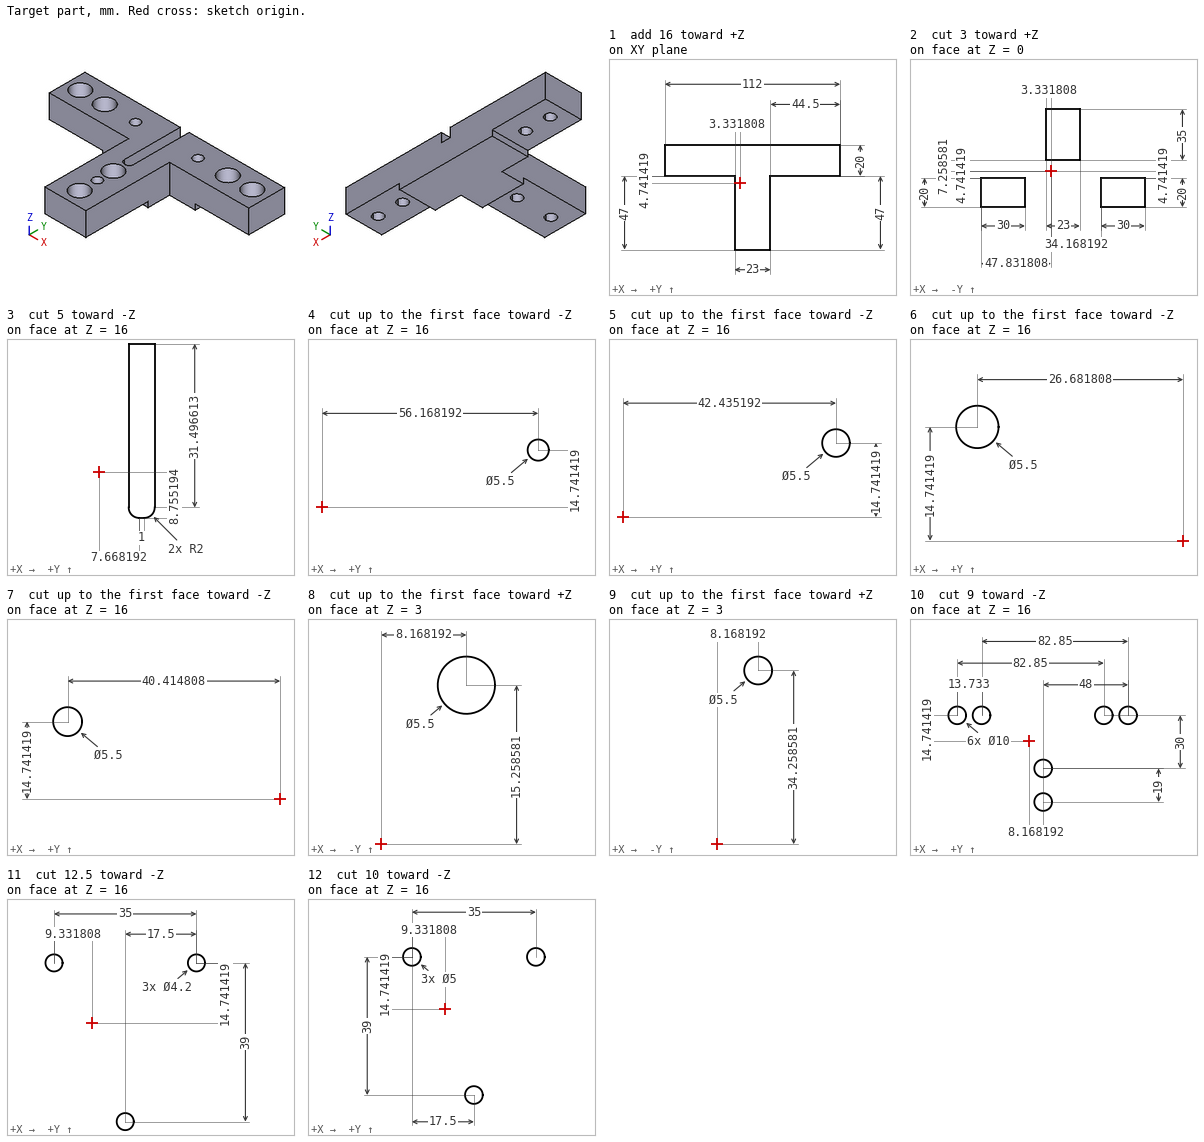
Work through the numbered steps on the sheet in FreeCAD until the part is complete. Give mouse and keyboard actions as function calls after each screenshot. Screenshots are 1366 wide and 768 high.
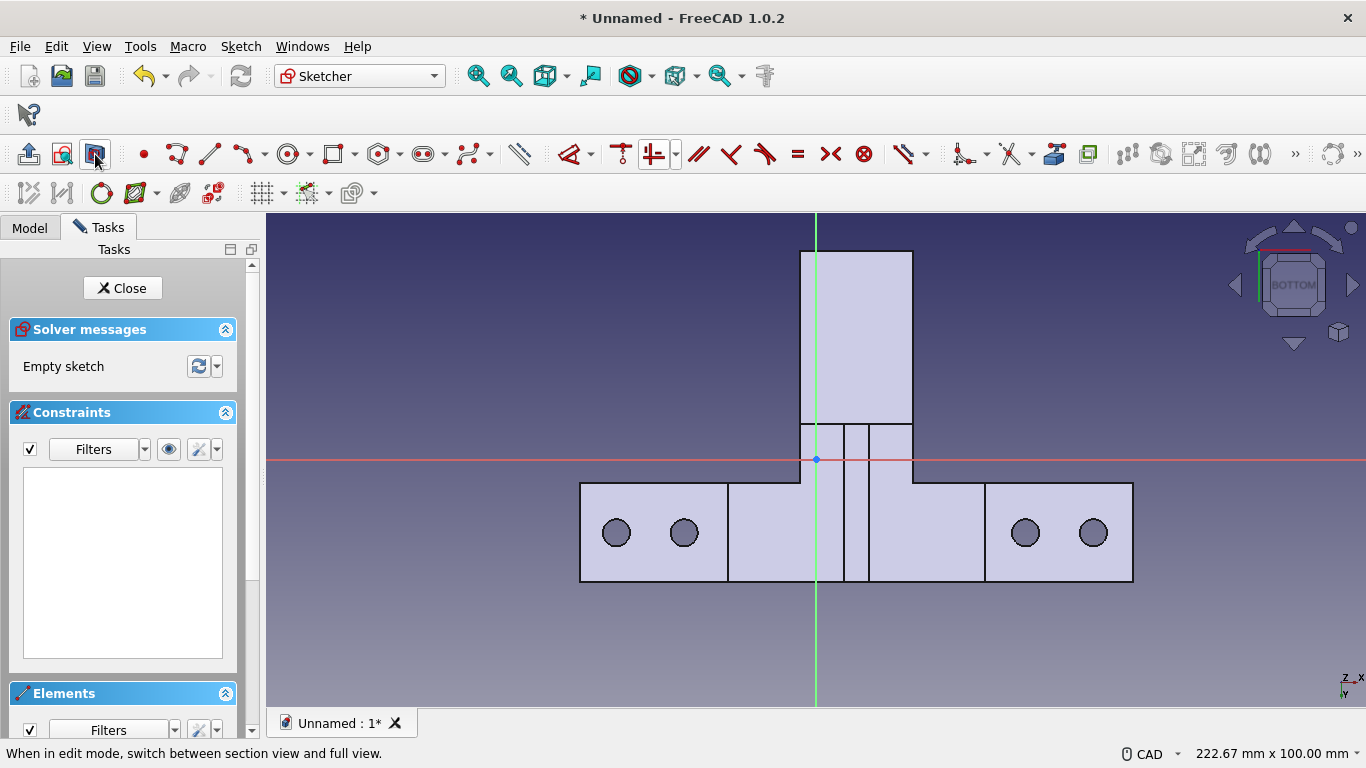
scroll(867, 377, up, 12)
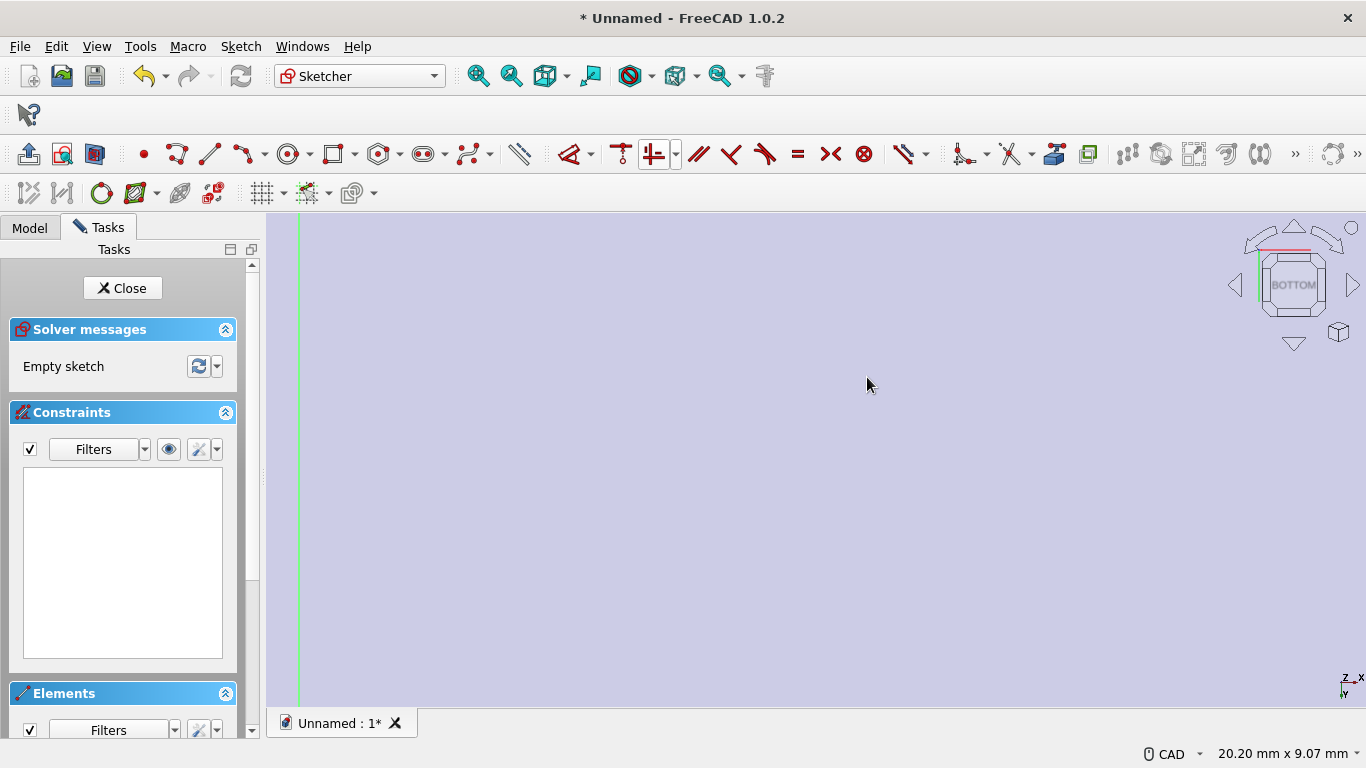
click(288, 154)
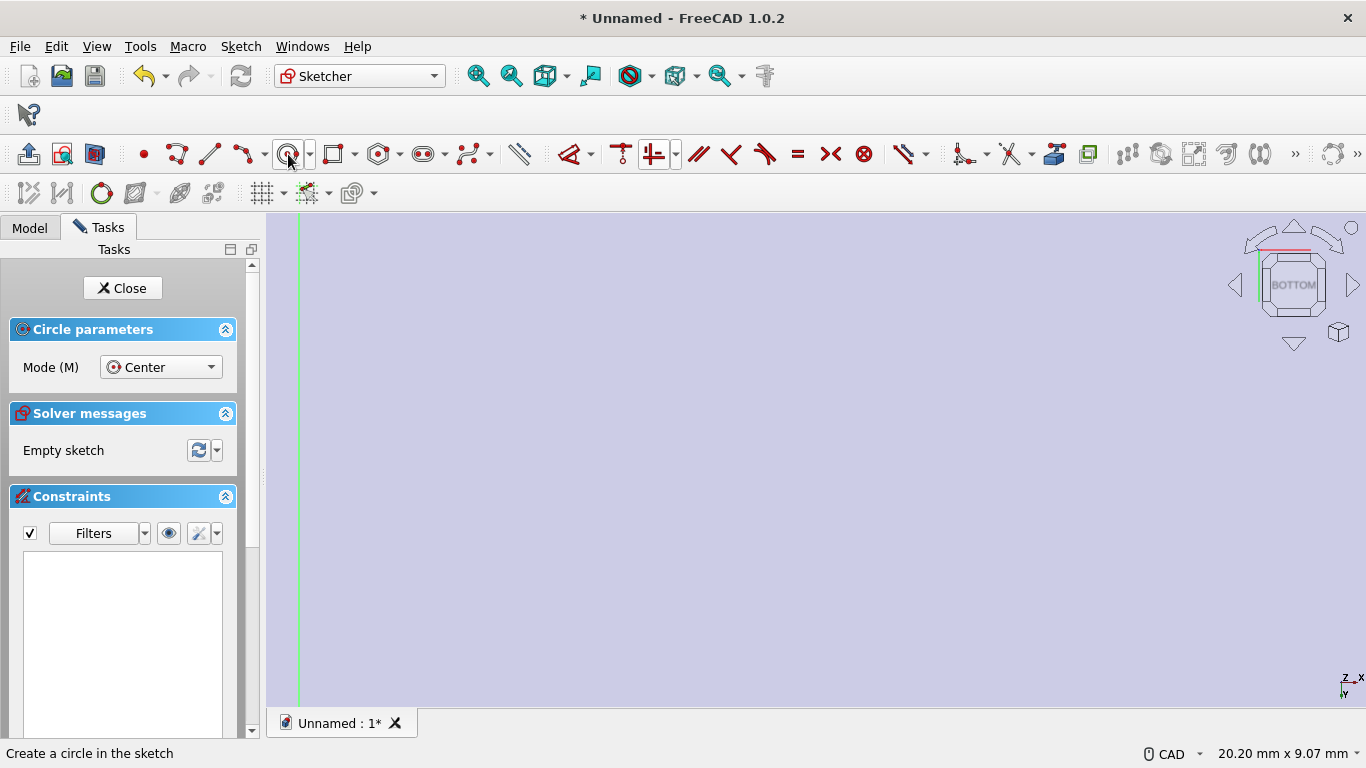
click(744, 458)
move(850, 352)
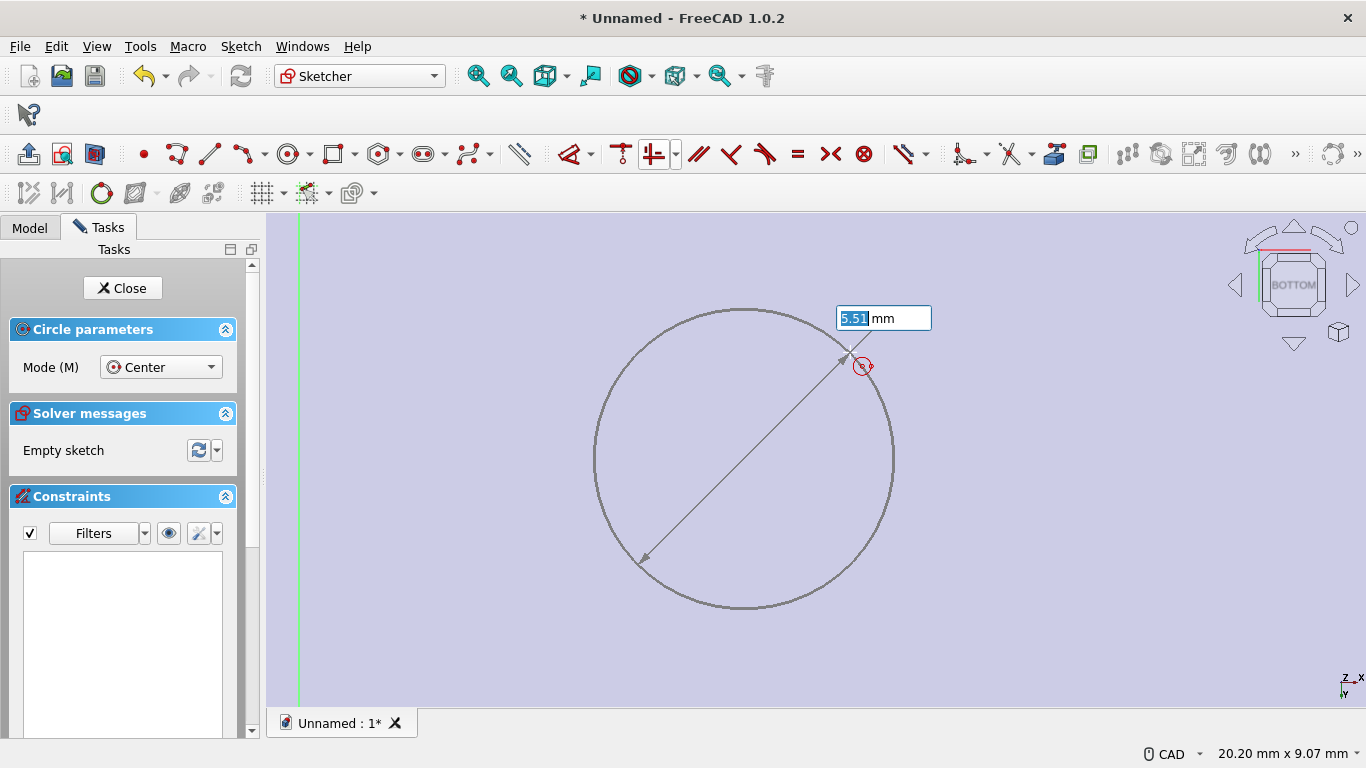
text(5.5)
key(Return)
key(Escape)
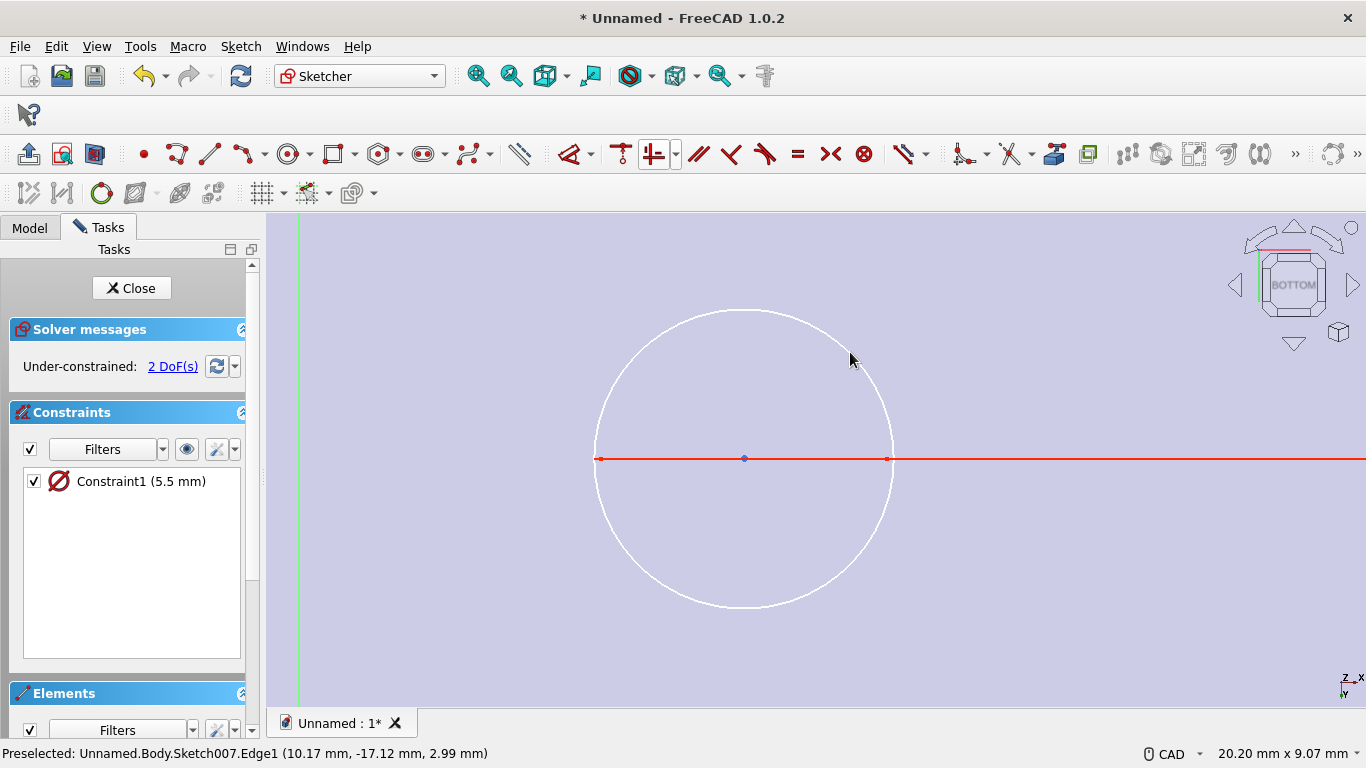
click(568, 154)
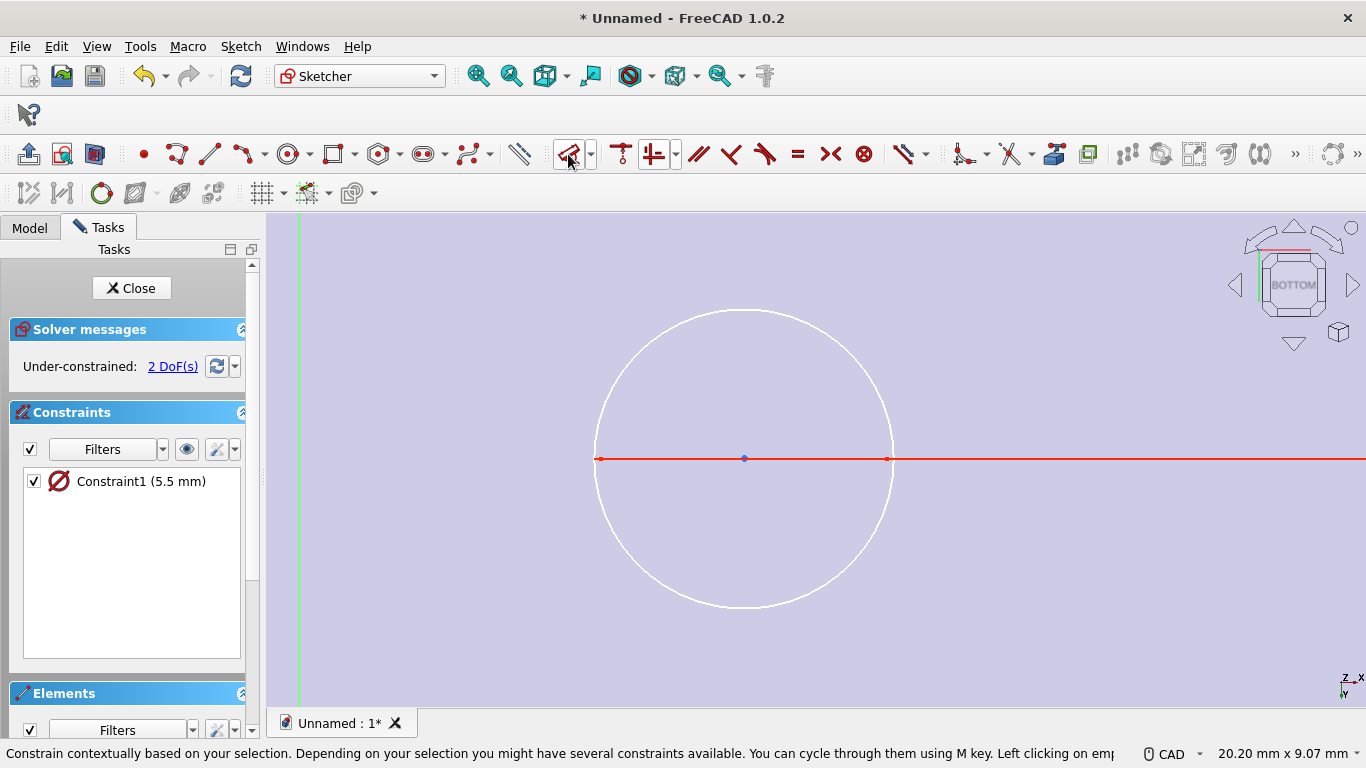
click(744, 459)
click(522, 425)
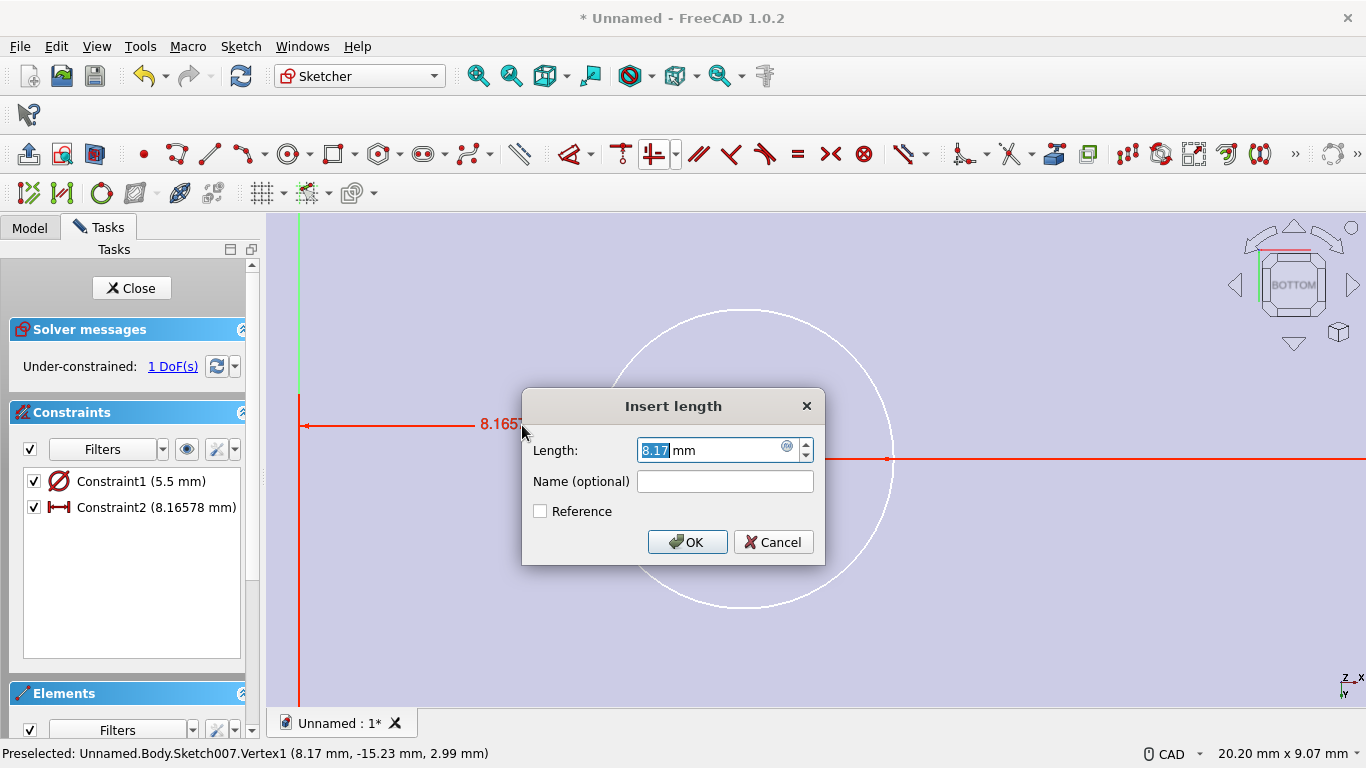
text(8.168192)
key(Return)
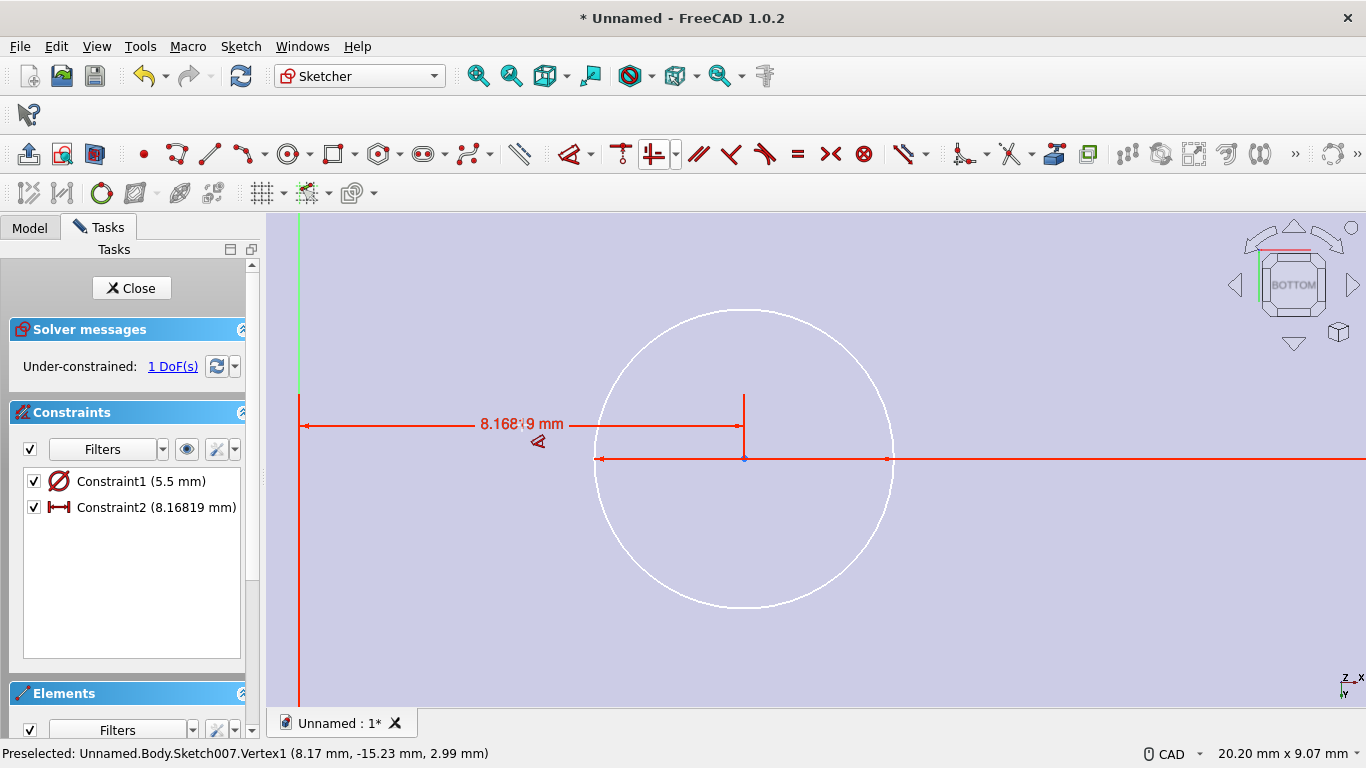
click(744, 459)
click(778, 569)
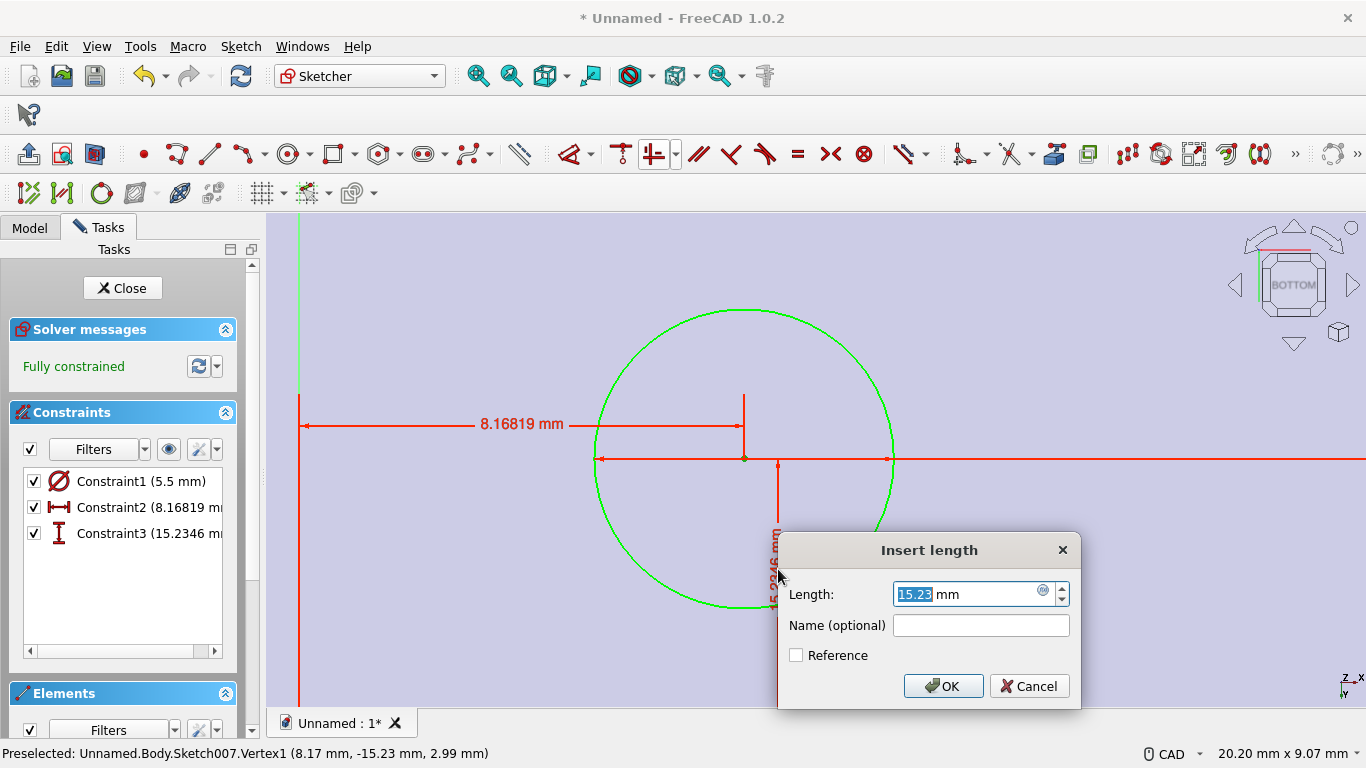
text(15.258581)
key(Return)
key(Escape)